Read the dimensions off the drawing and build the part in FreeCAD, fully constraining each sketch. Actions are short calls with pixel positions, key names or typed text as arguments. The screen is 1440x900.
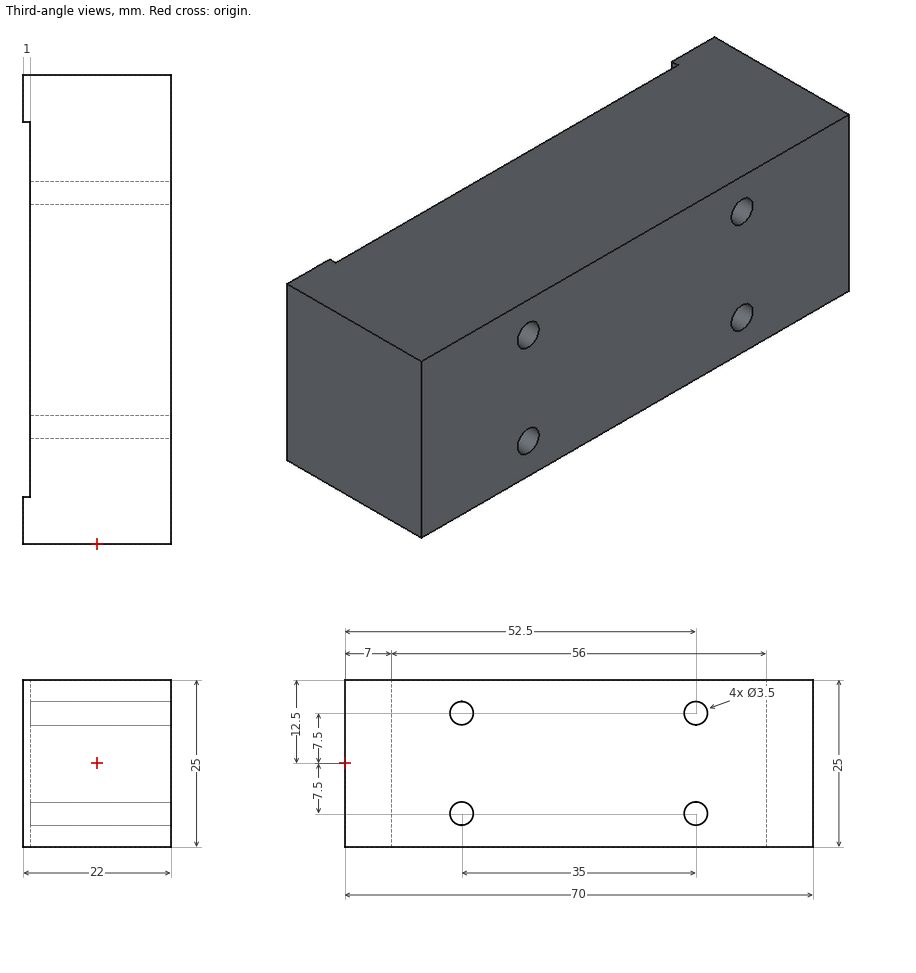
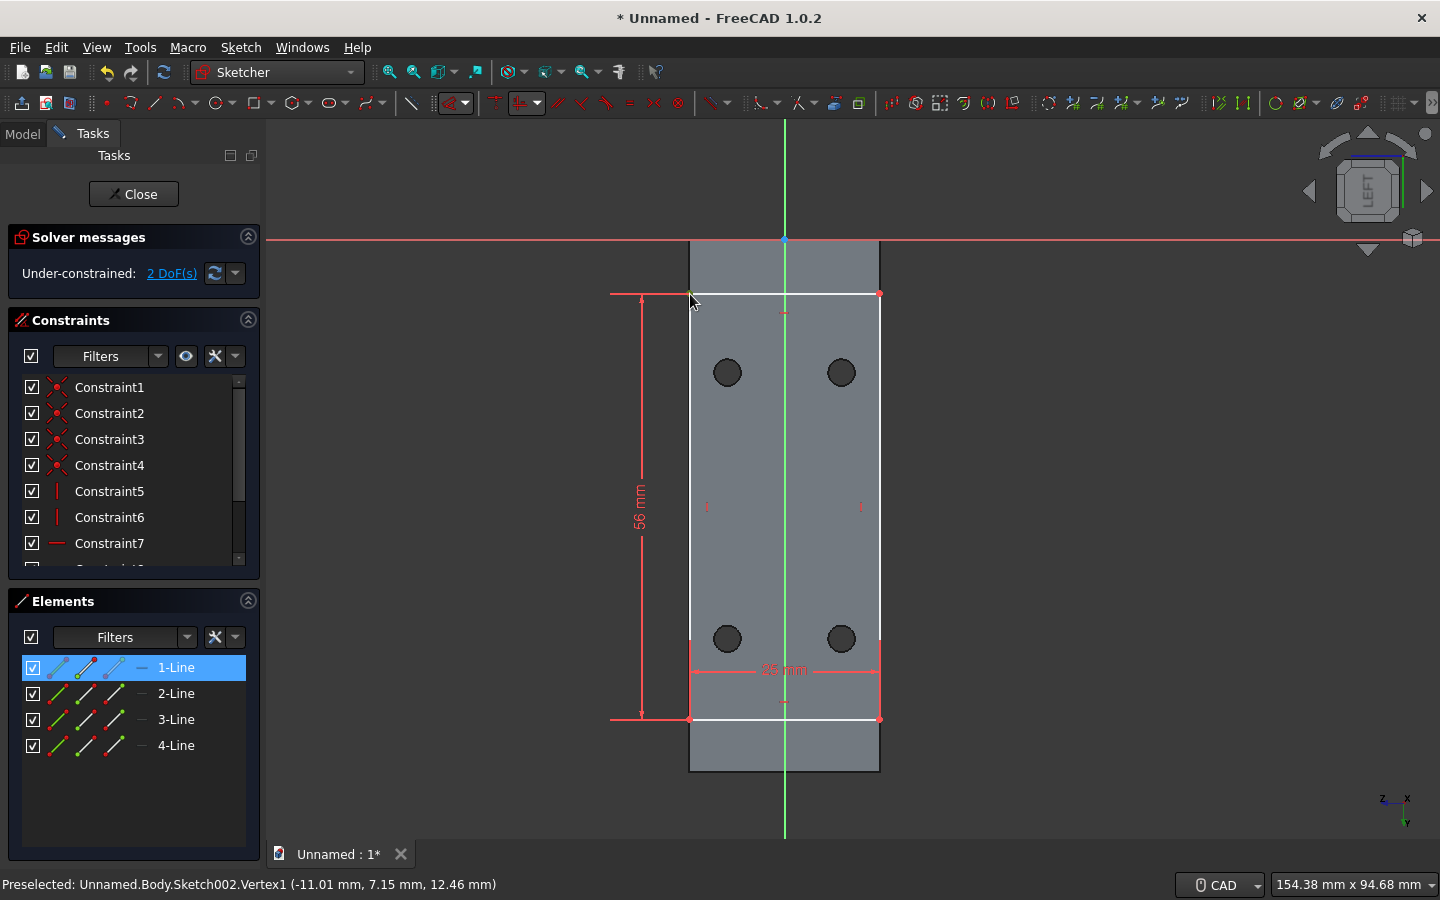
key(i)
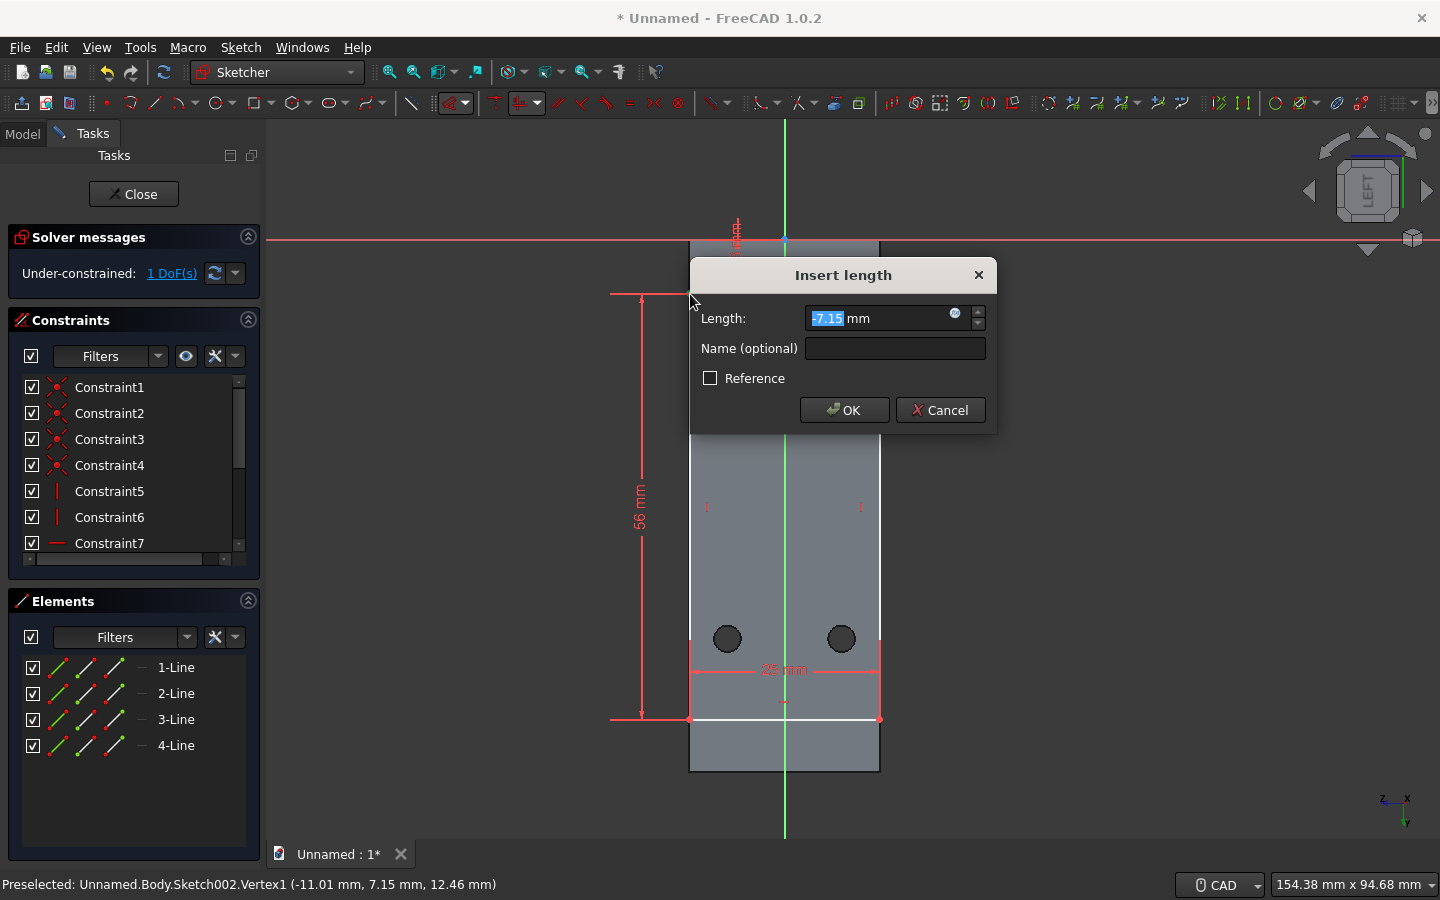
text(-7)
key(Return)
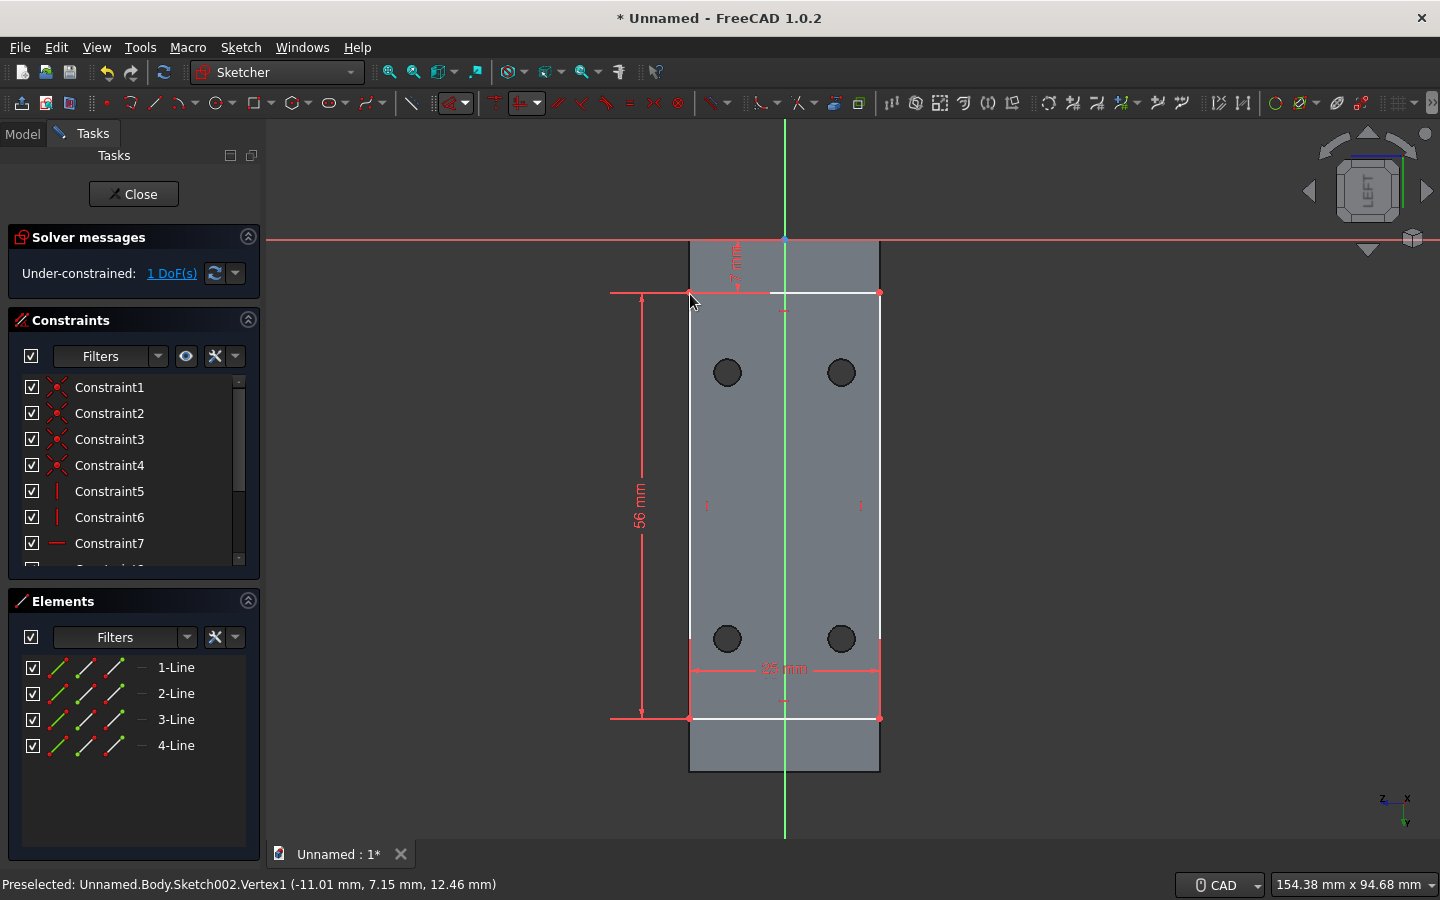
click(690, 293)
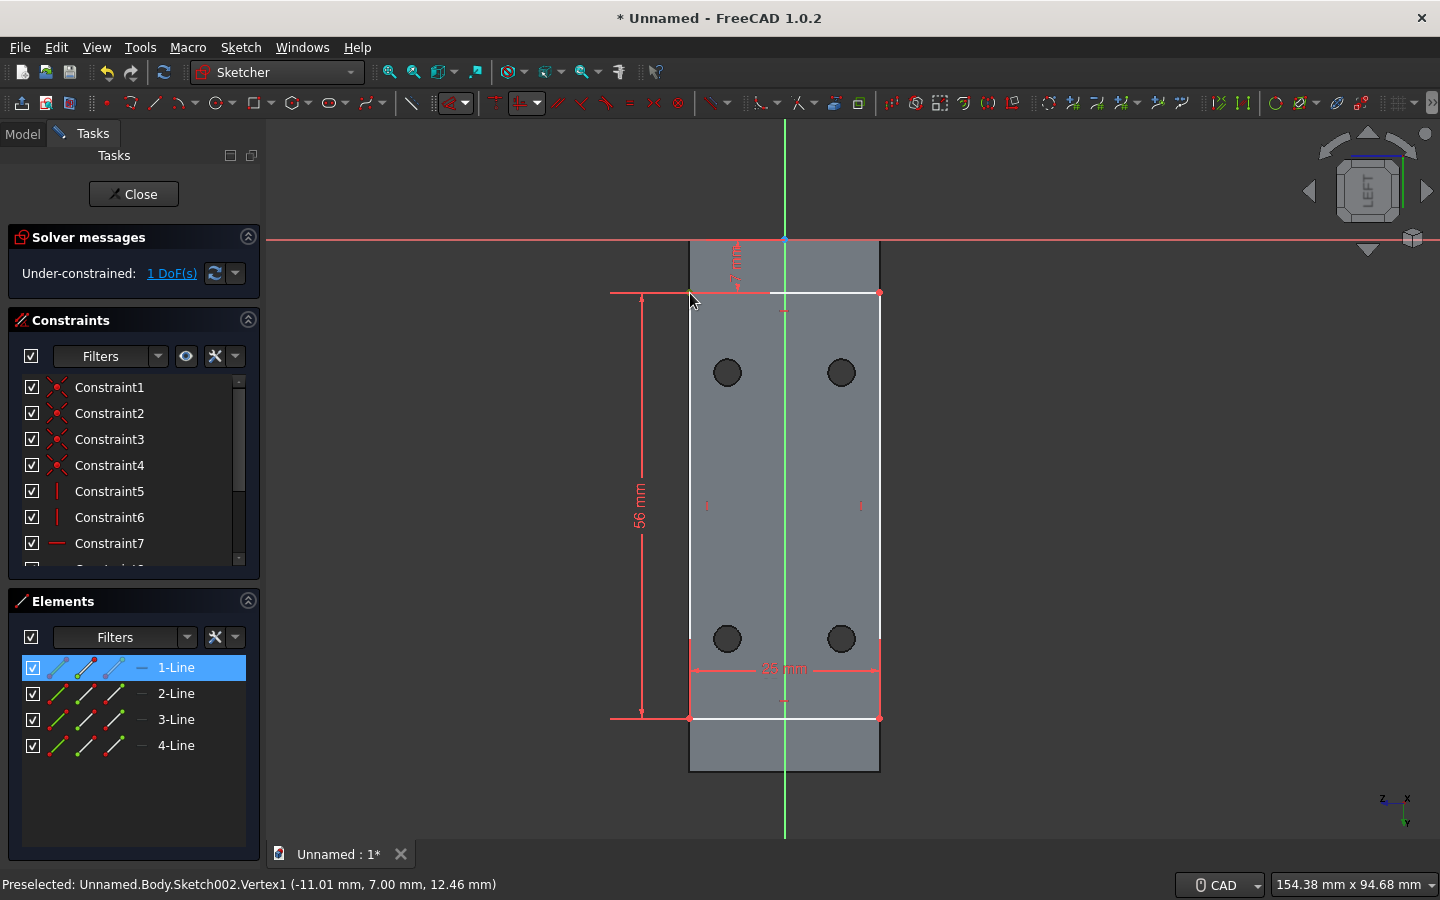
click(468, 104)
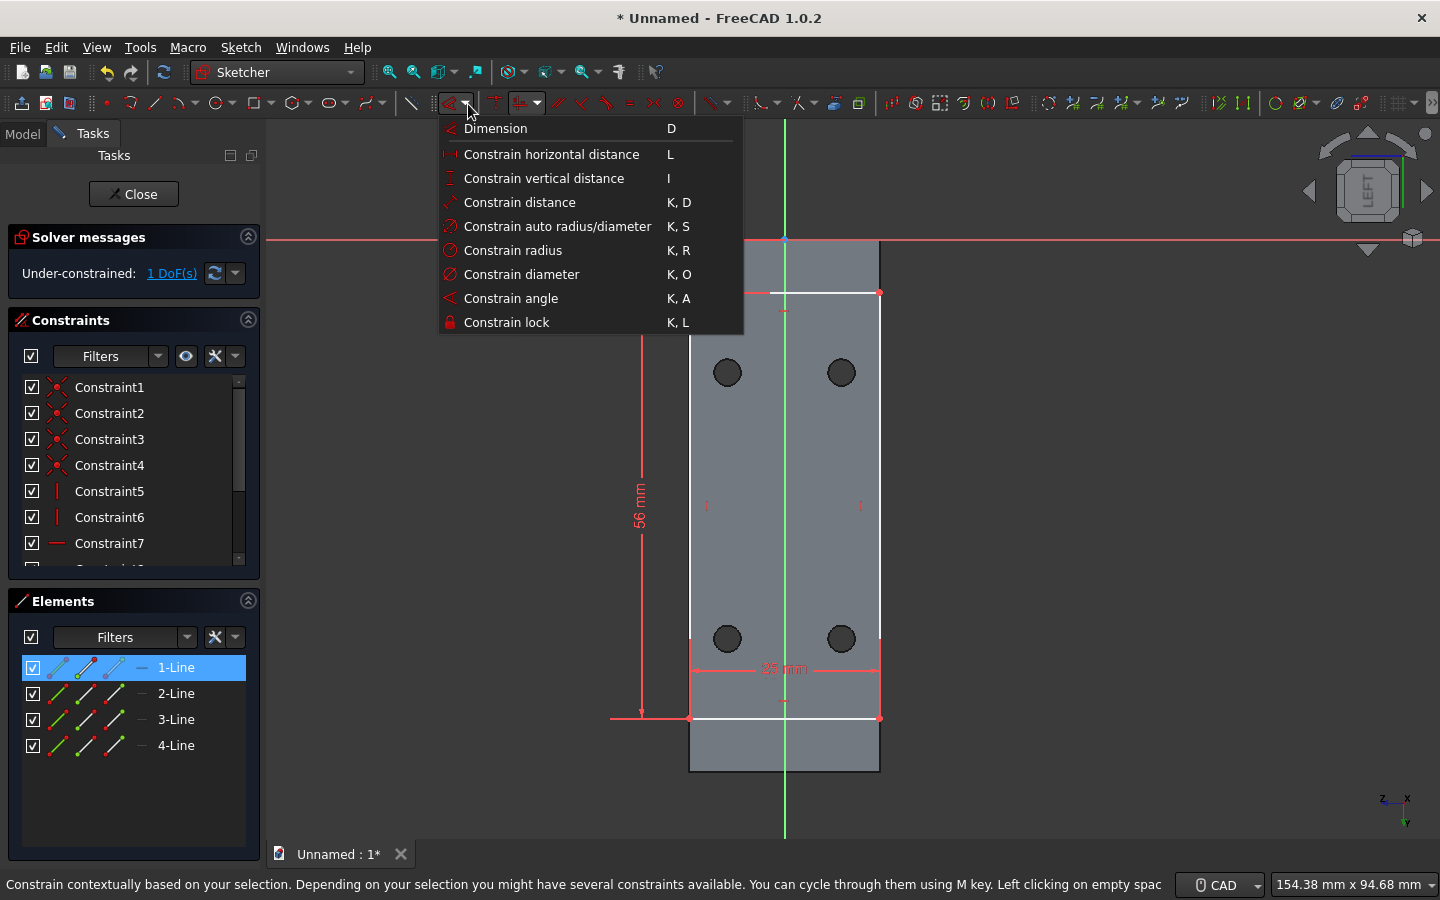
click(591, 154)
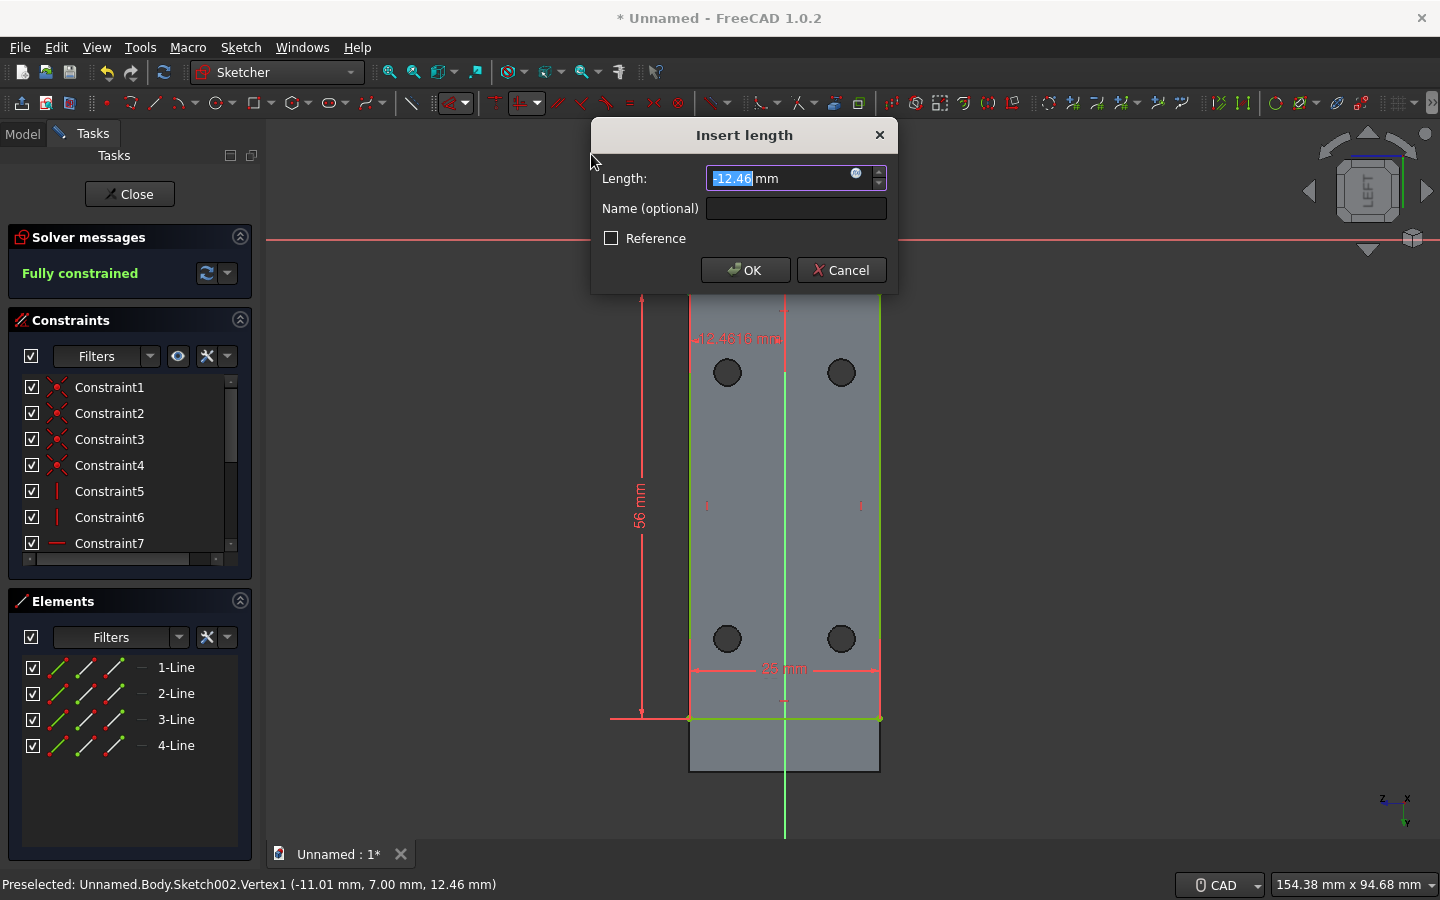
text(-12.5)
key(Return)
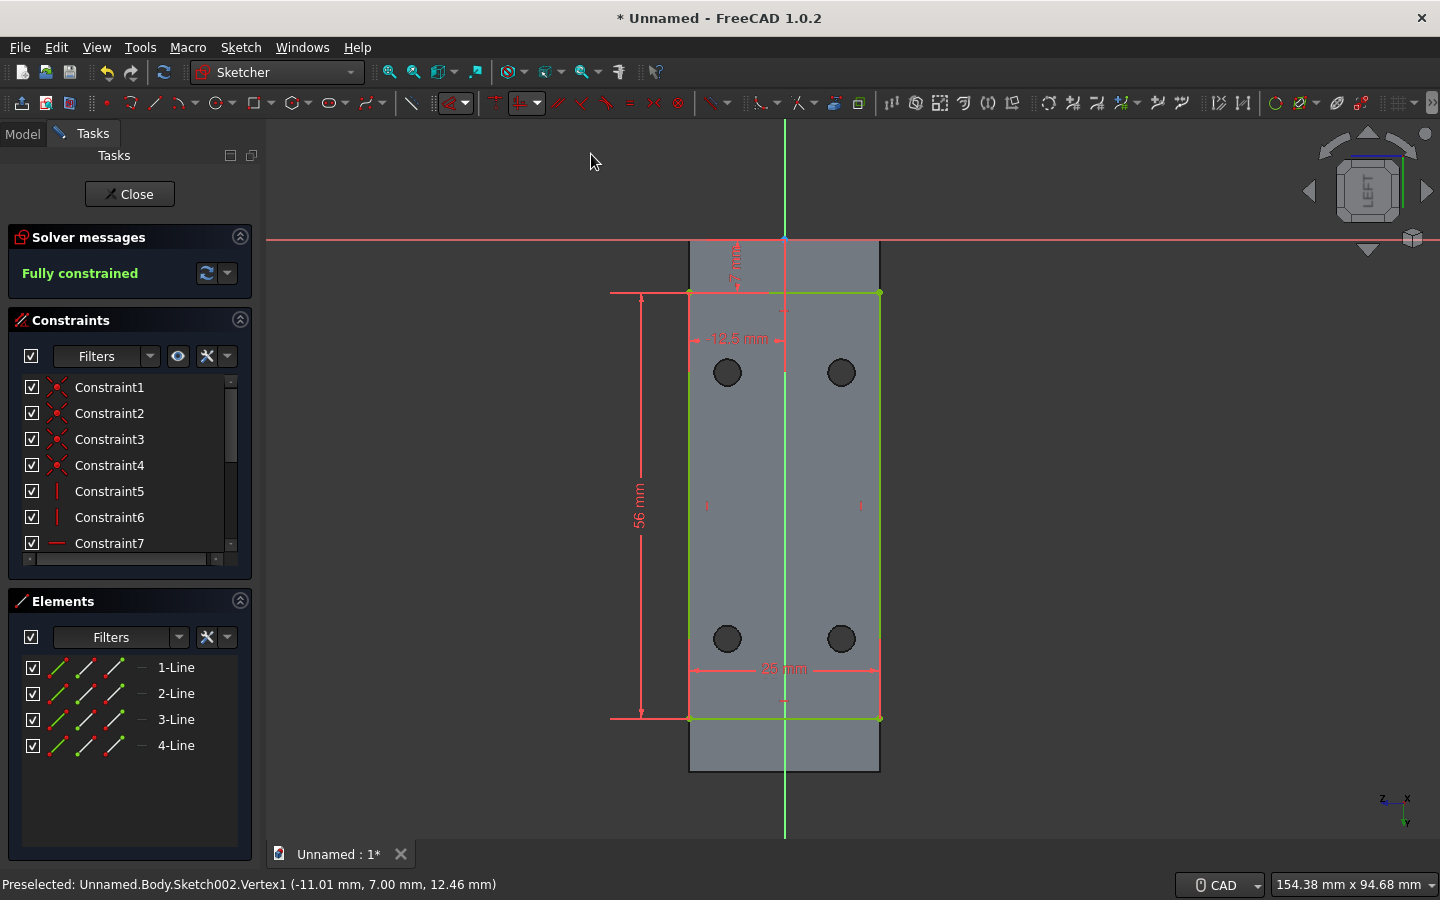
click(130, 194)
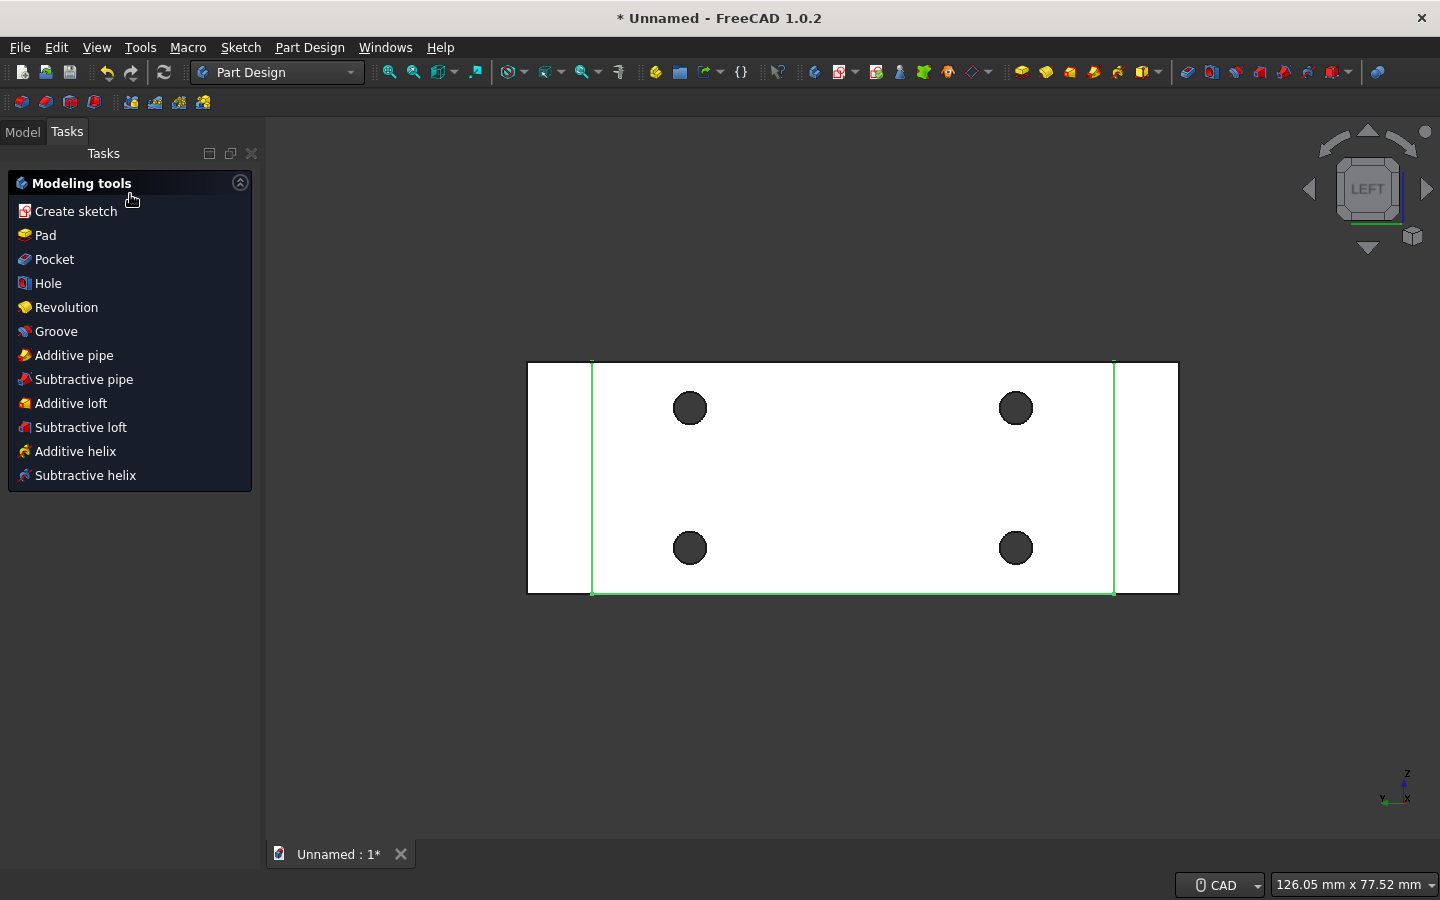
click(1188, 72)